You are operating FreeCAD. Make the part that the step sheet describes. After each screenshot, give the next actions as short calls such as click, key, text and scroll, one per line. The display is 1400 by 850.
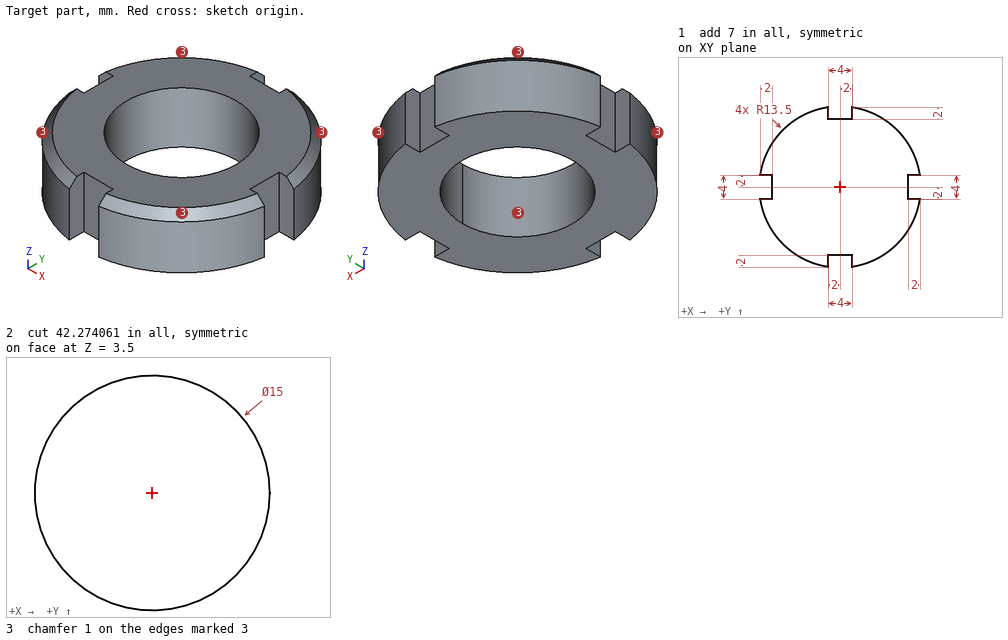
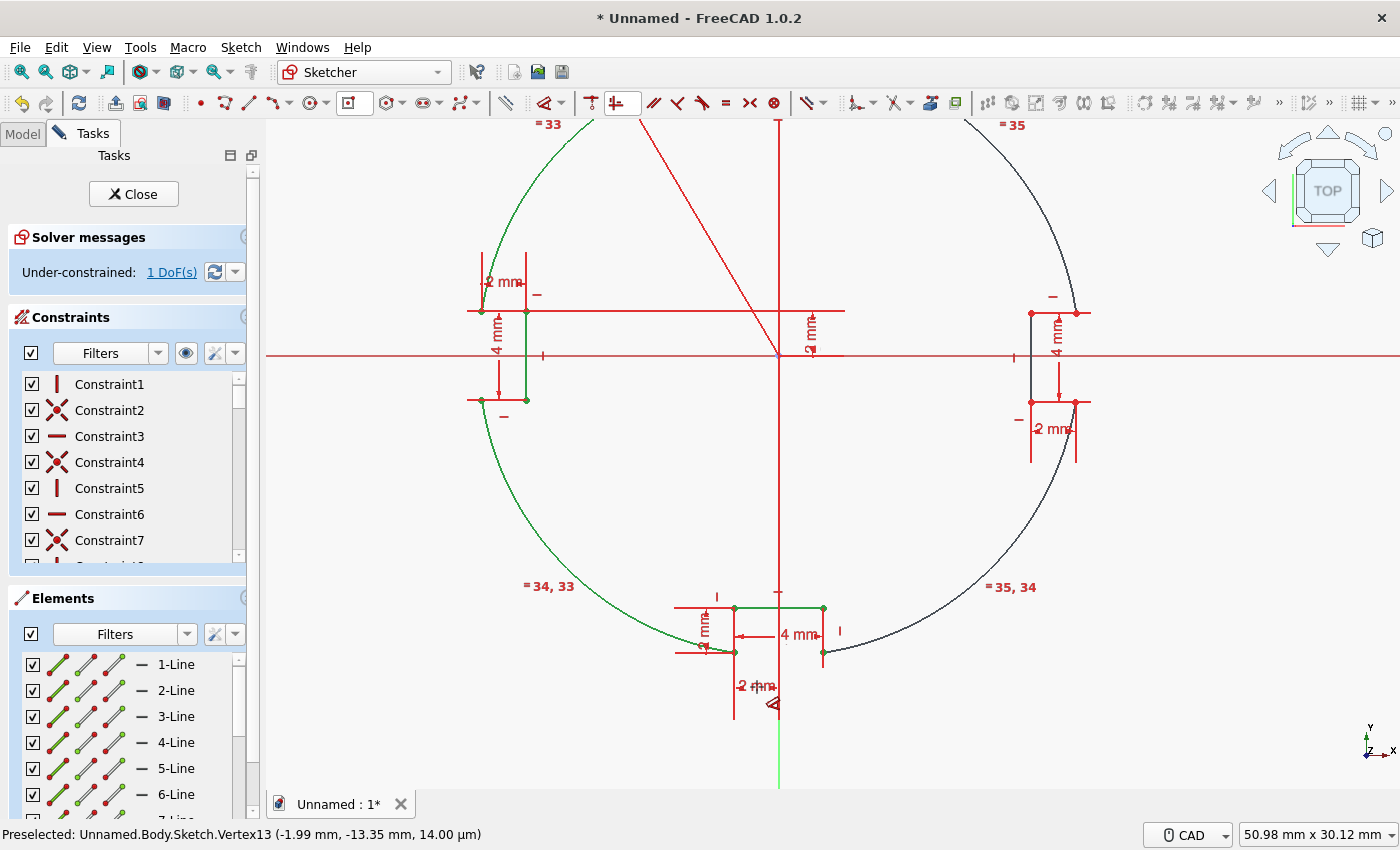
click(1076, 402)
click(1110, 379)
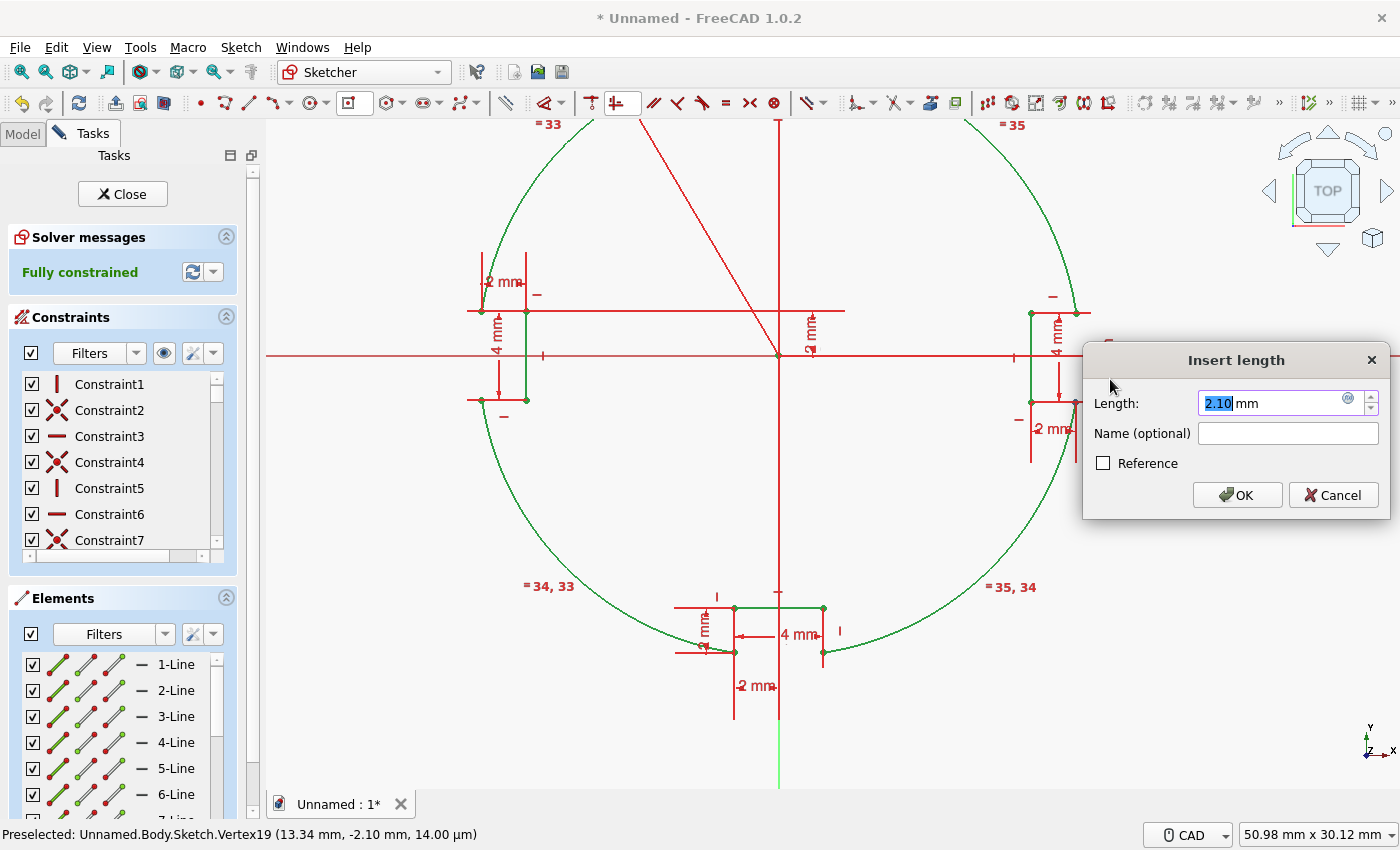
text(2)
key(Return)
key(Escape)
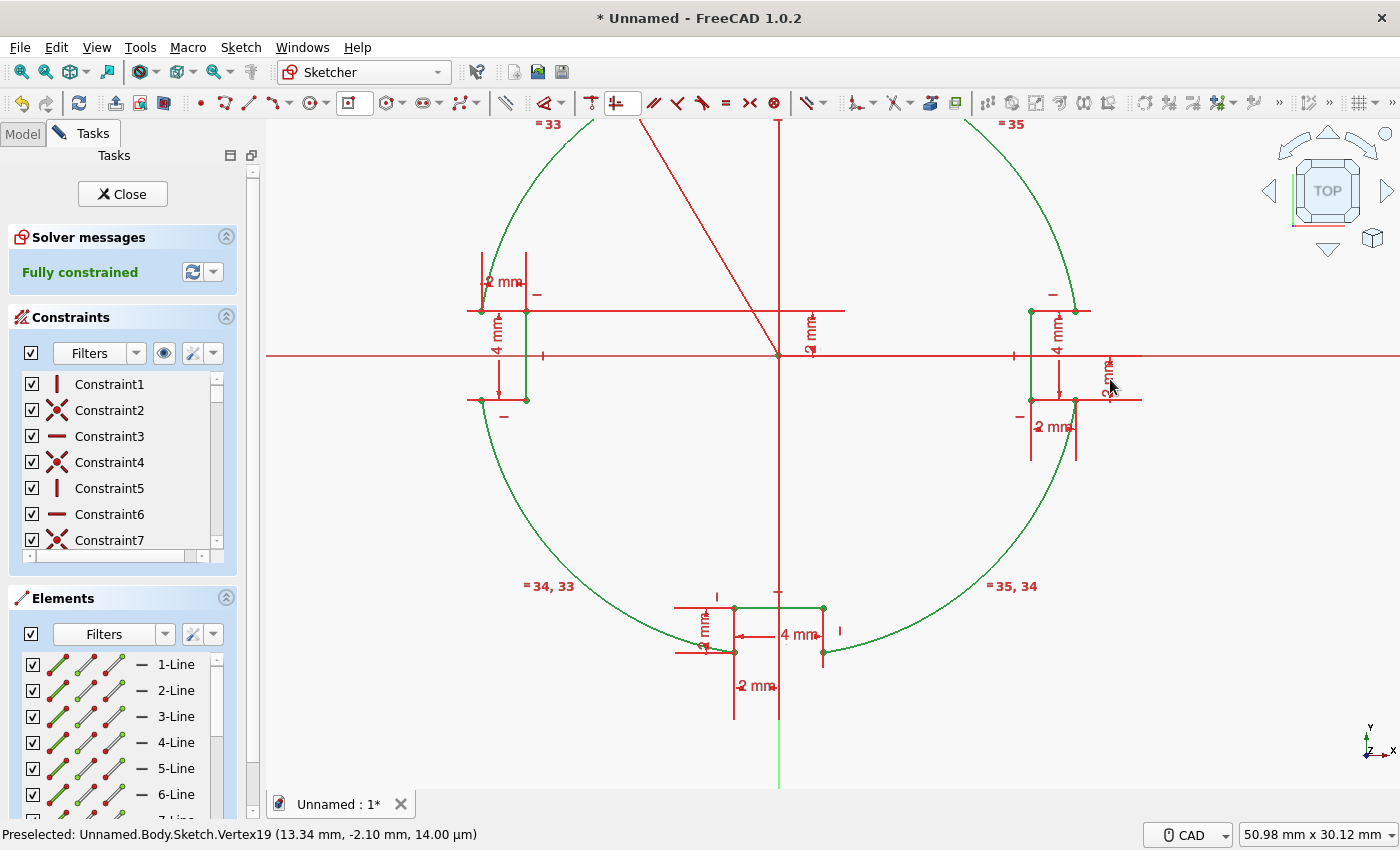
click(123, 194)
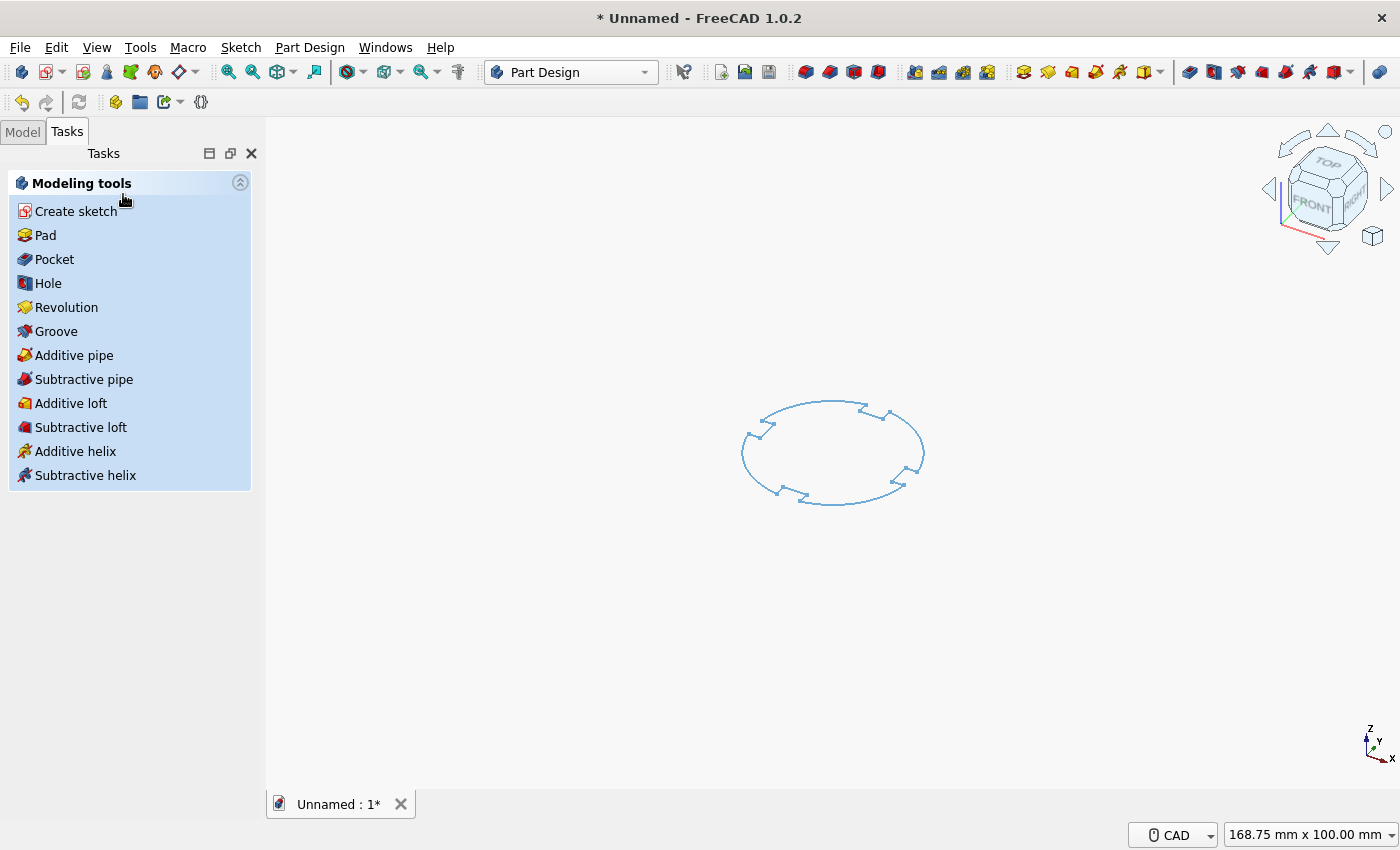
click(1024, 72)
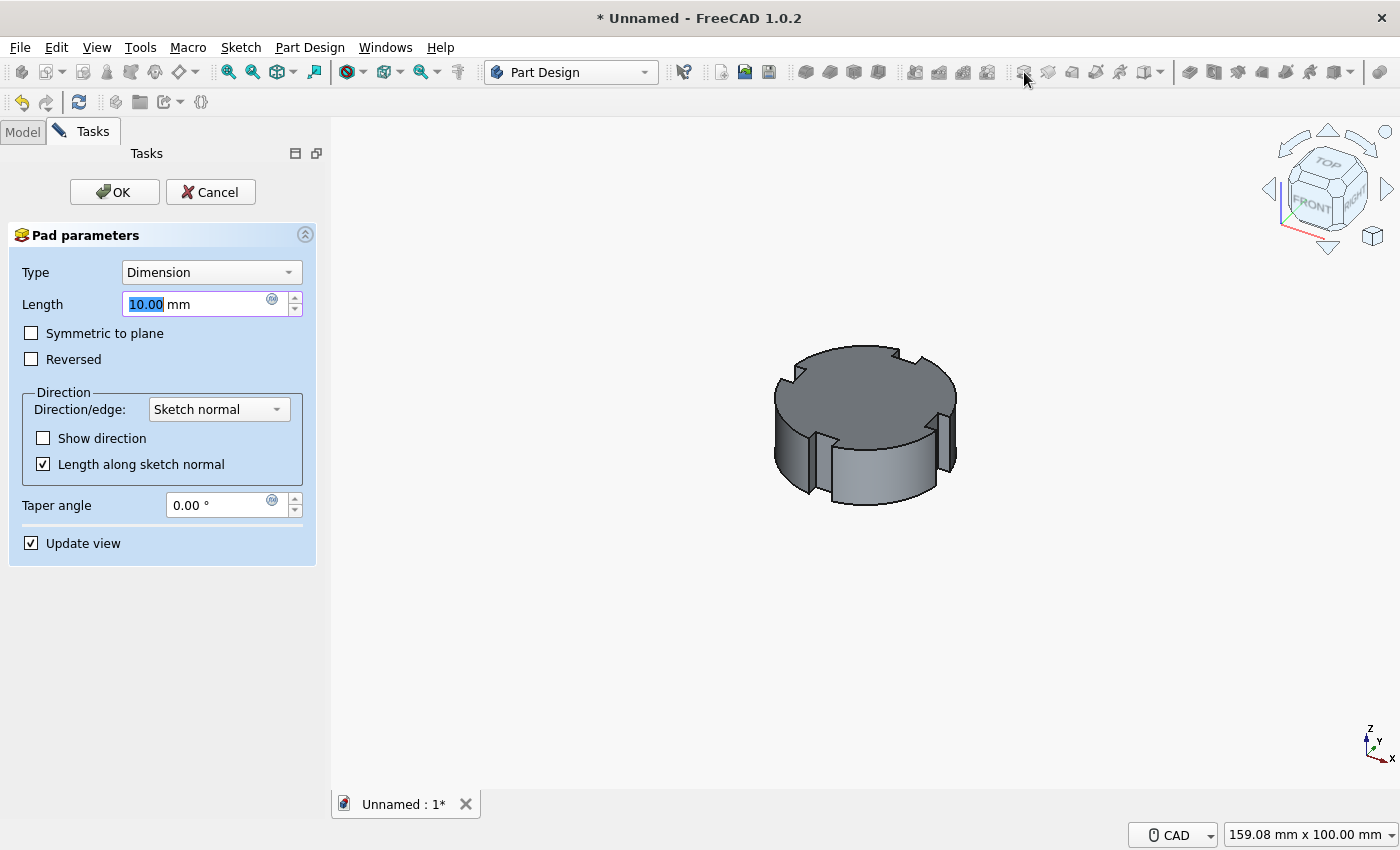
text(7)
key(Tab)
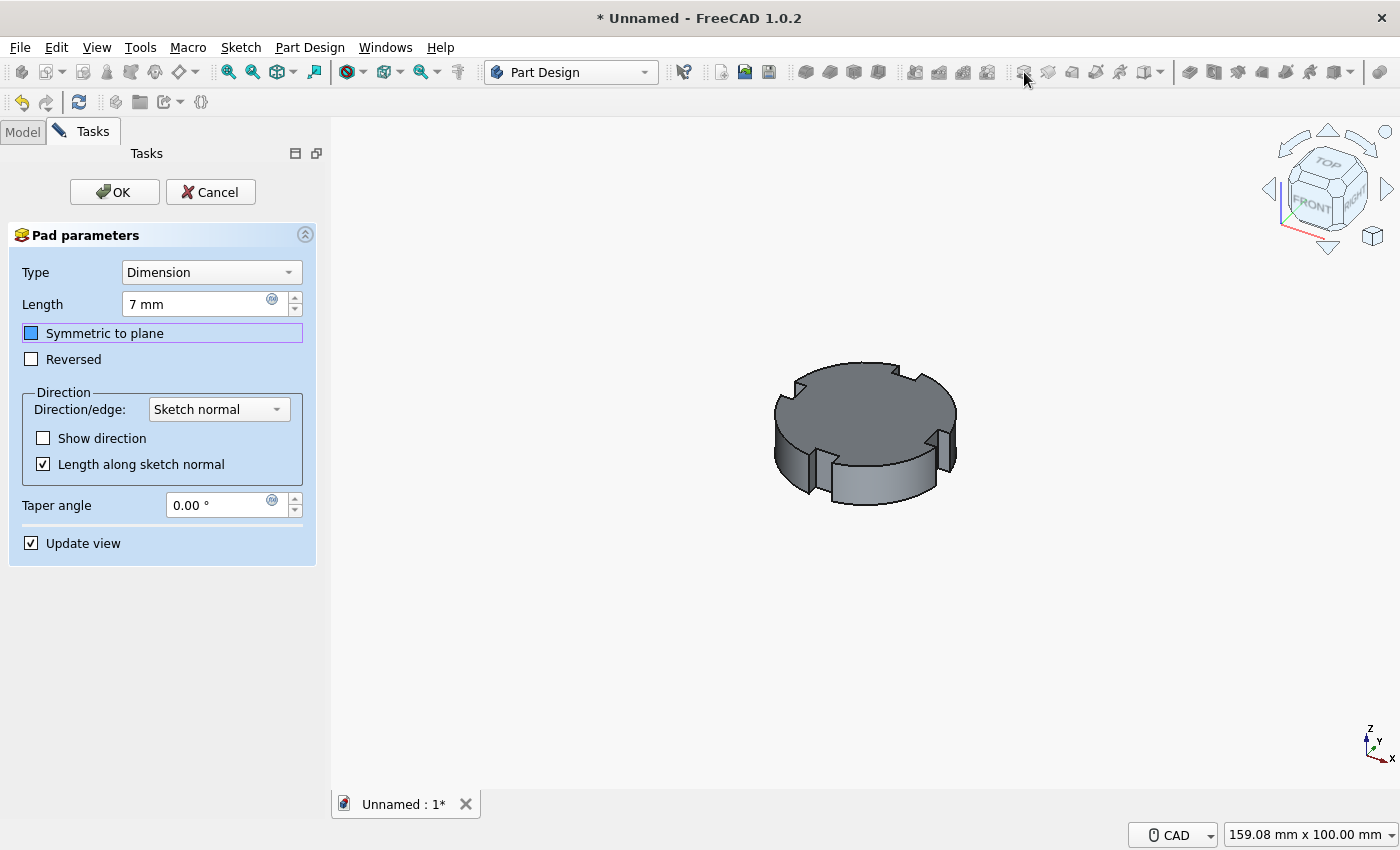
click(30, 333)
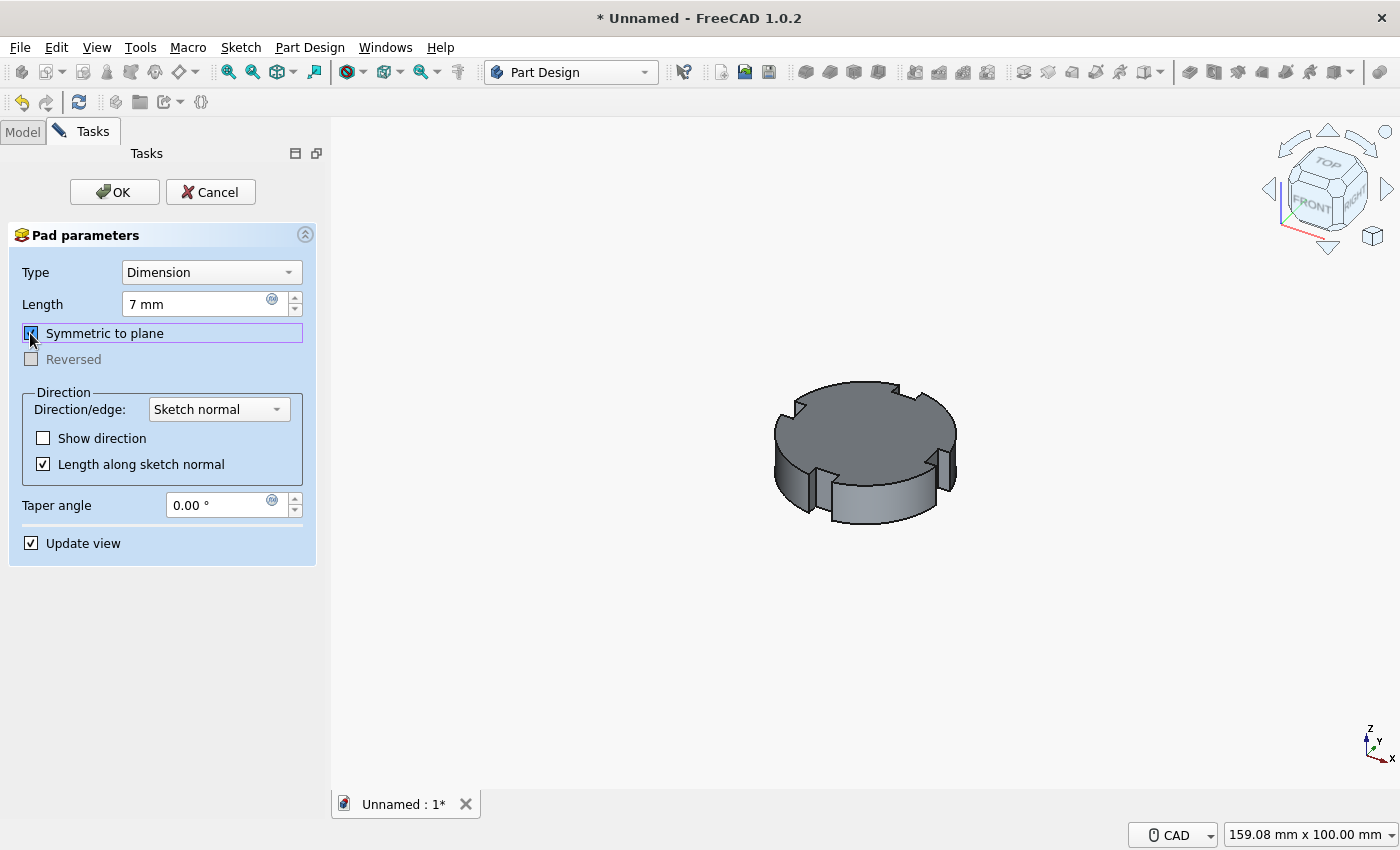
click(115, 192)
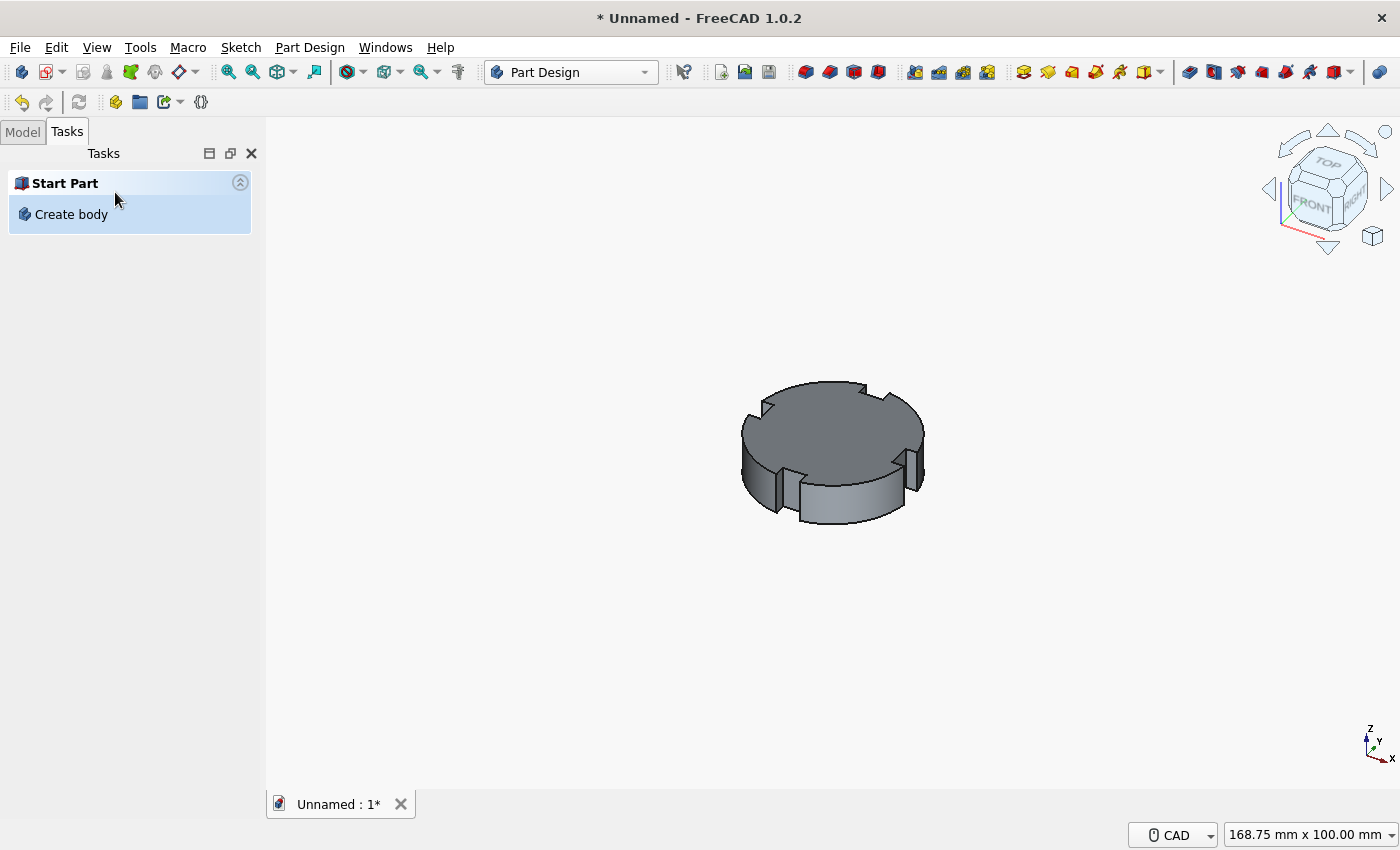
key(v)
key(f)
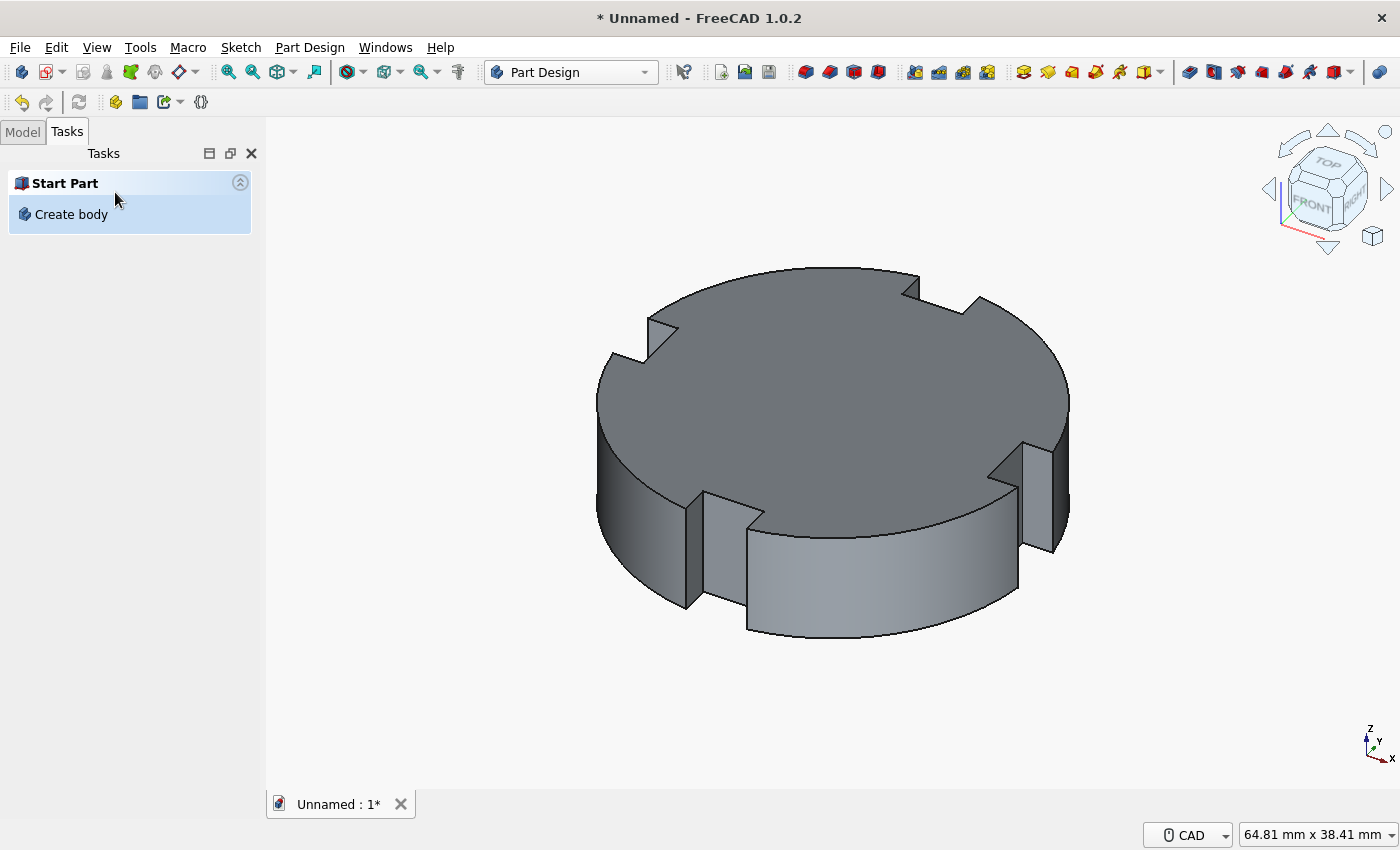
click(833, 402)